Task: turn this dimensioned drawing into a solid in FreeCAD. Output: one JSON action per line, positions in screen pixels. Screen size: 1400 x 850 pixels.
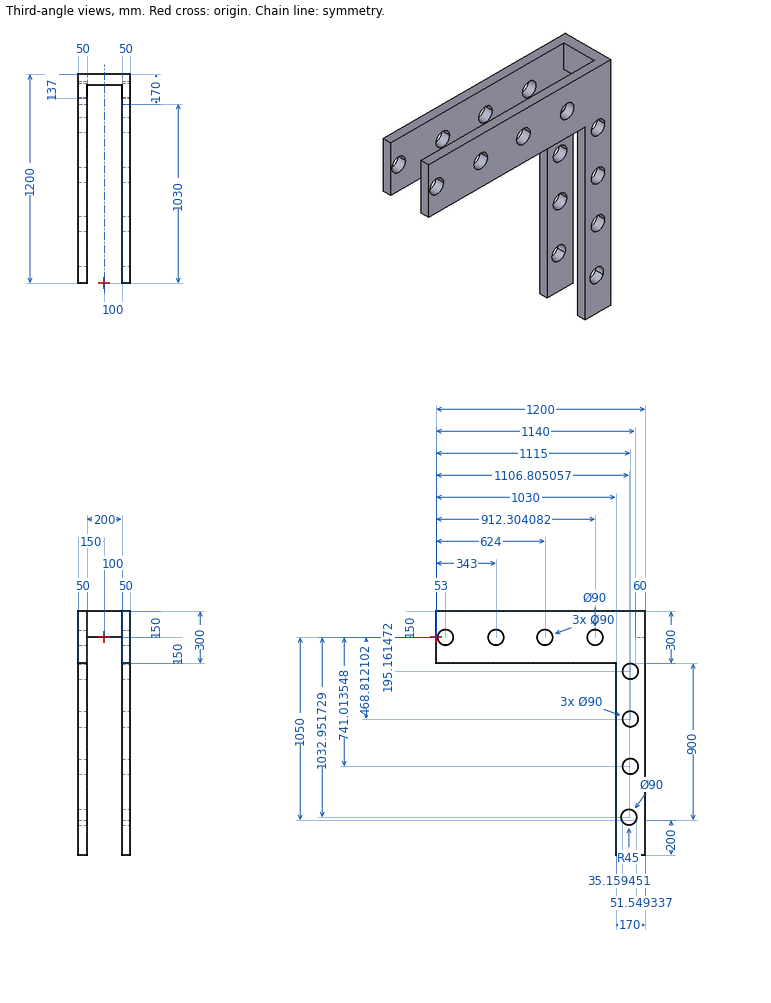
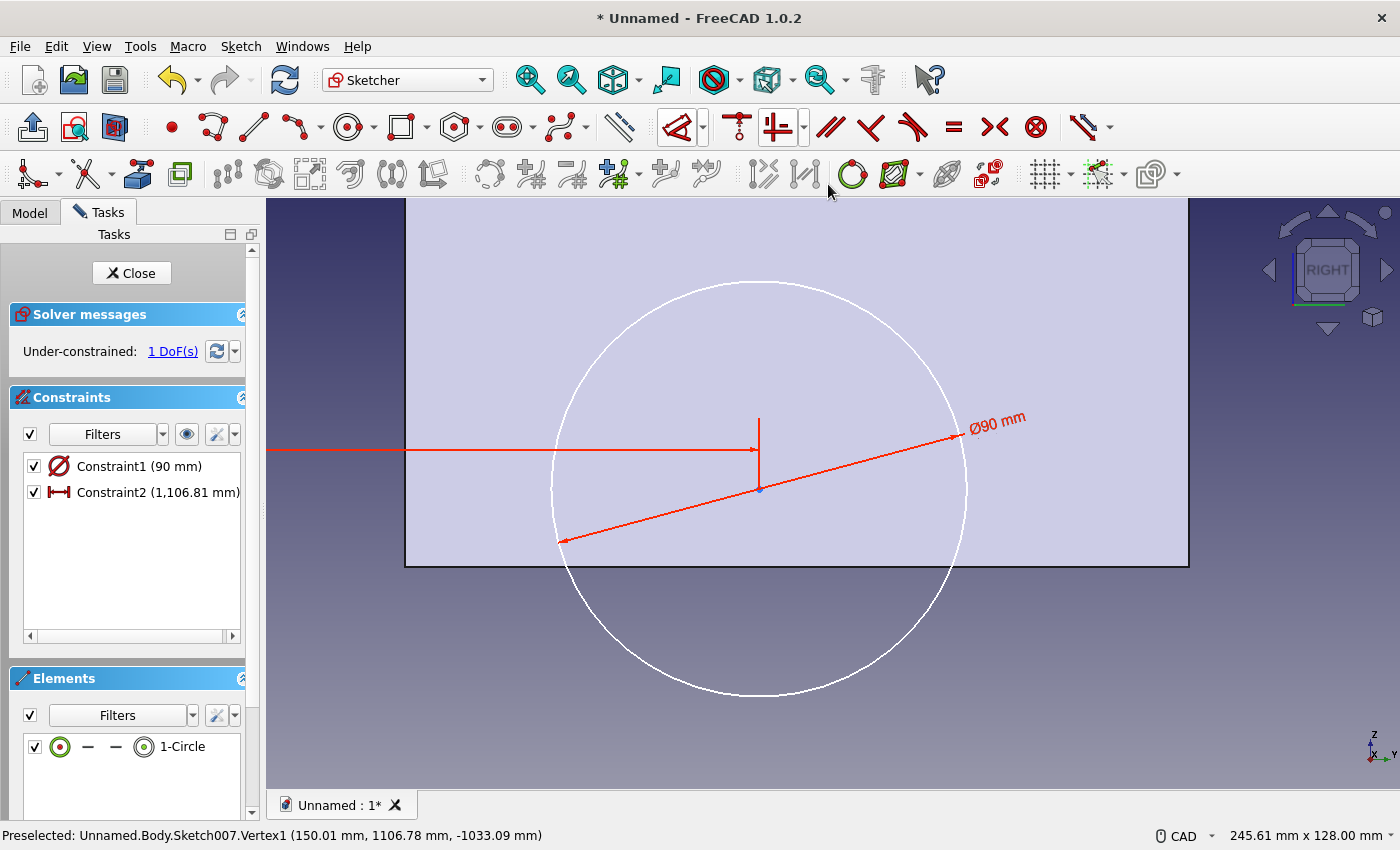
{"action": "left_click", "coordinate": [759, 489]}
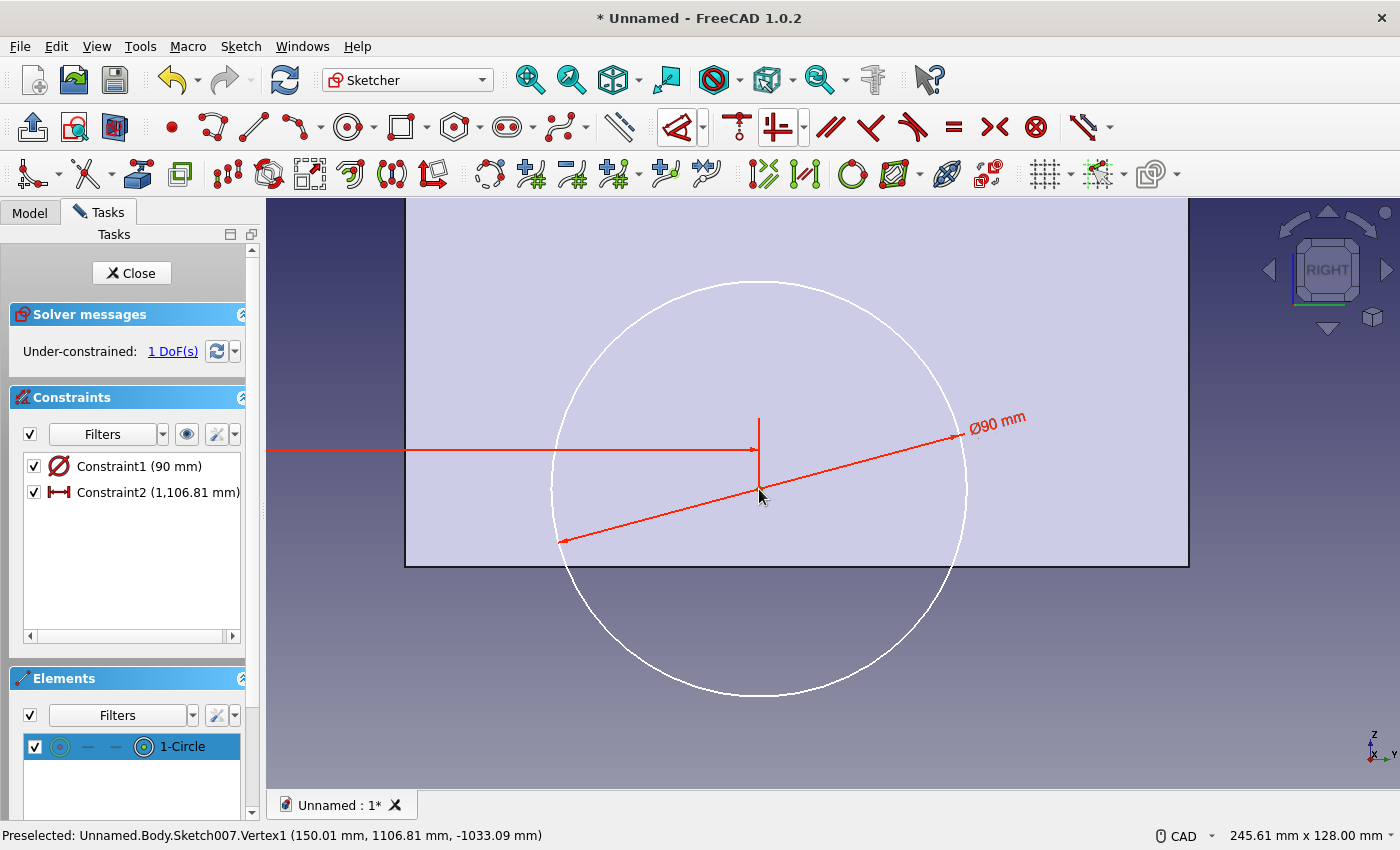
{"action": "left_click", "coordinate": [702, 128]}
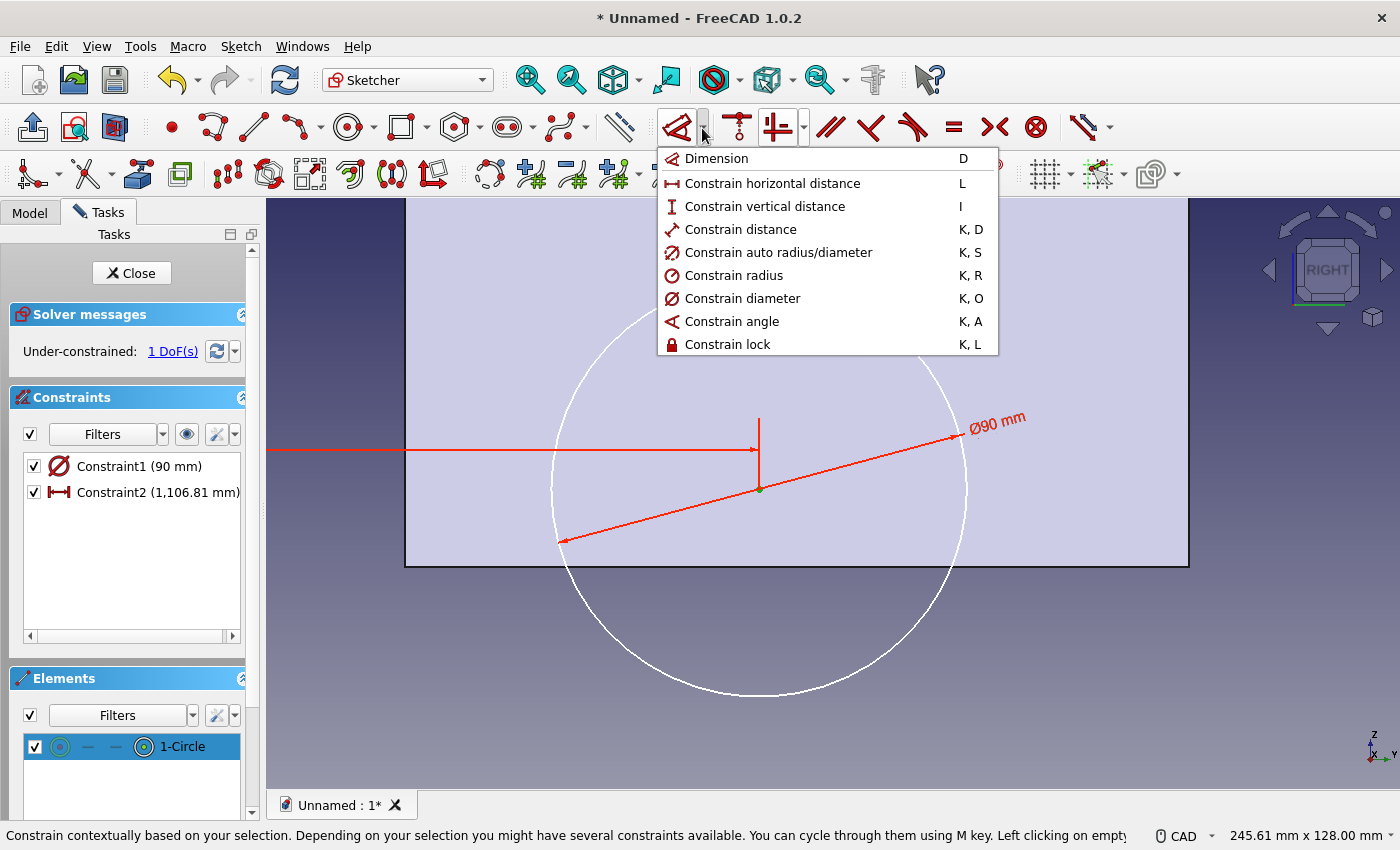
{"action": "left_click", "coordinate": [828, 206]}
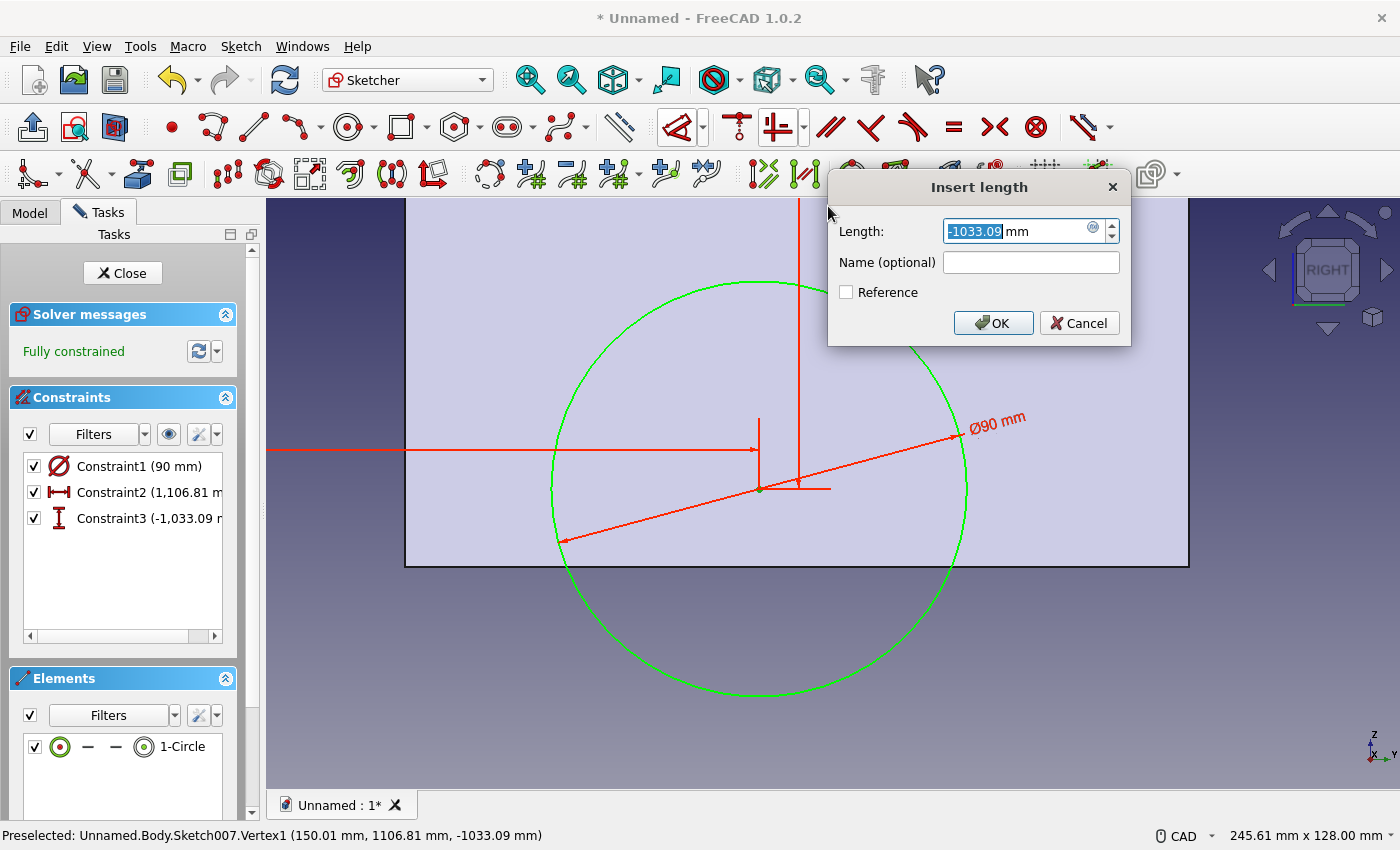
{"action": "type", "text": "-1032.951729"}
{"action": "key", "text": "Return"}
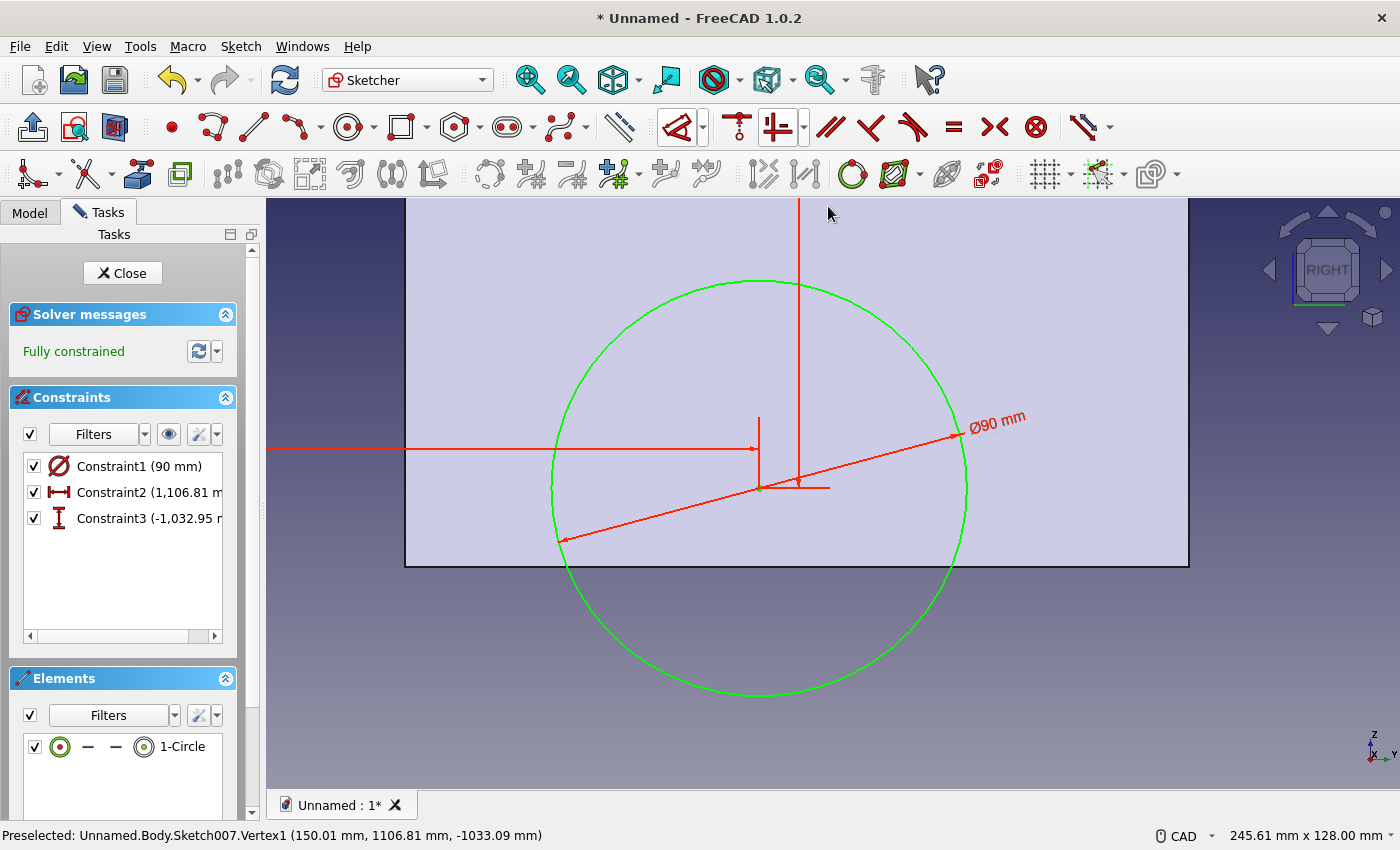
{"action": "left_click", "coordinate": [123, 273]}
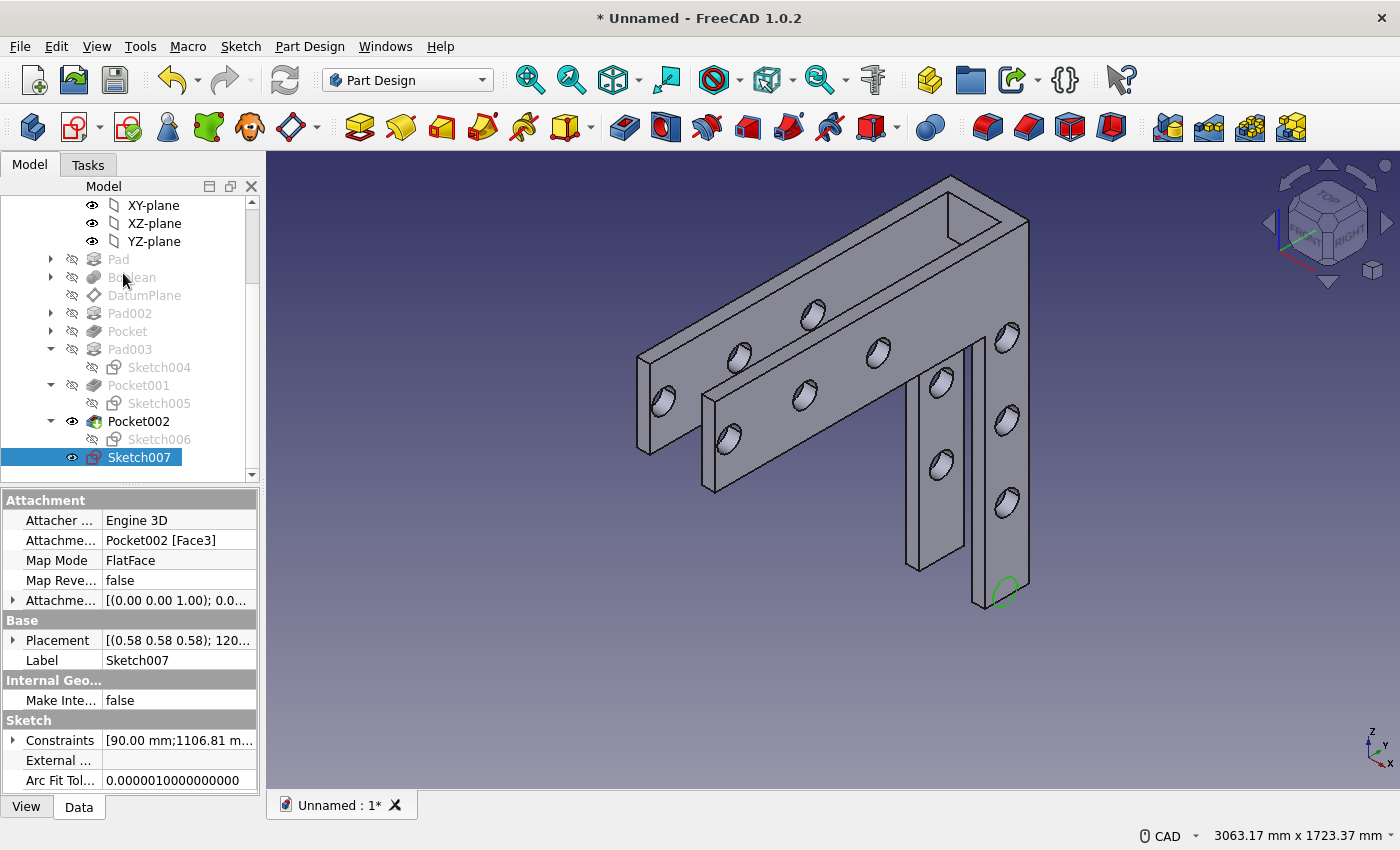
{"action": "left_click", "coordinate": [625, 128]}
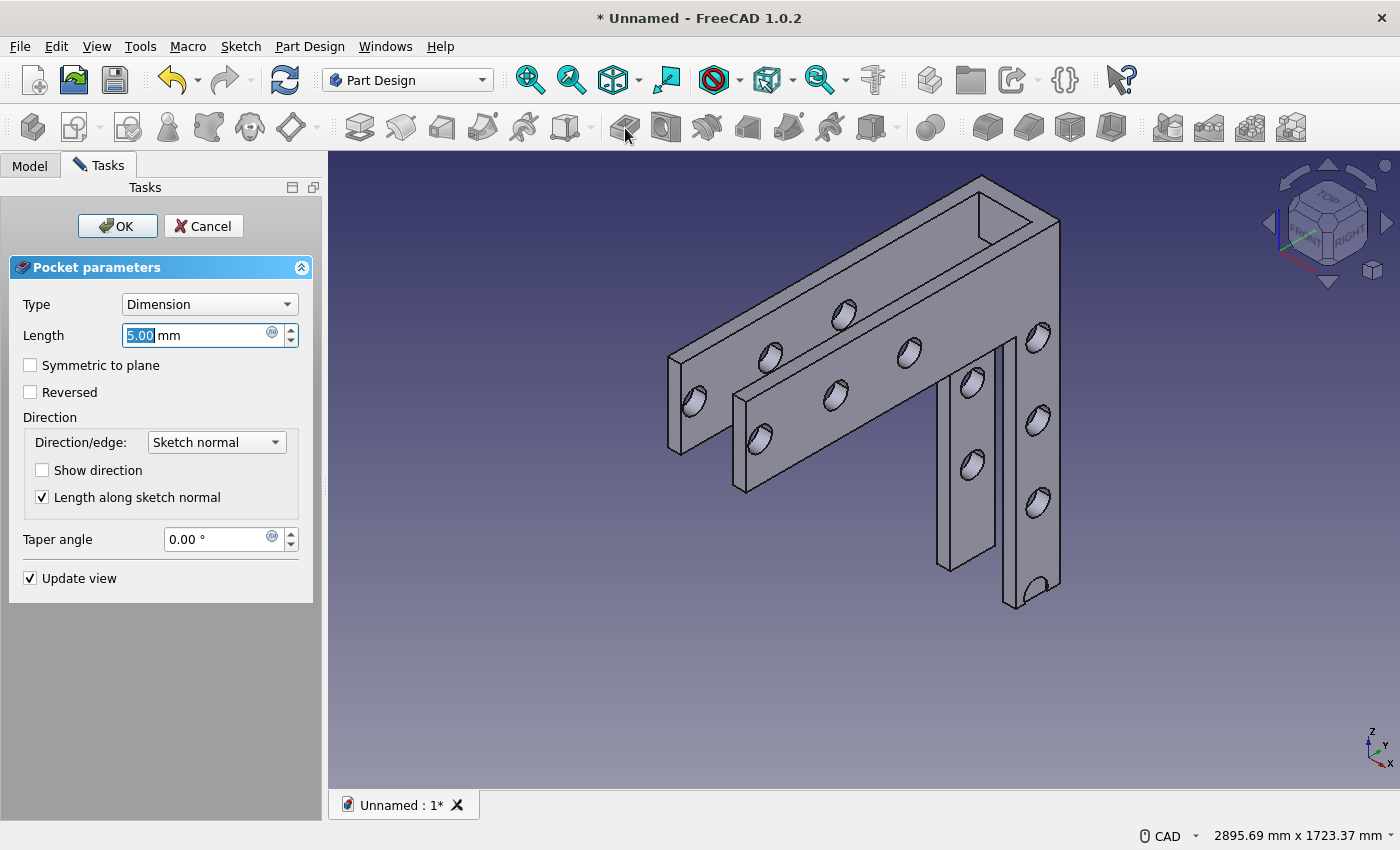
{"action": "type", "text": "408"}
{"action": "key", "text": "Tab"}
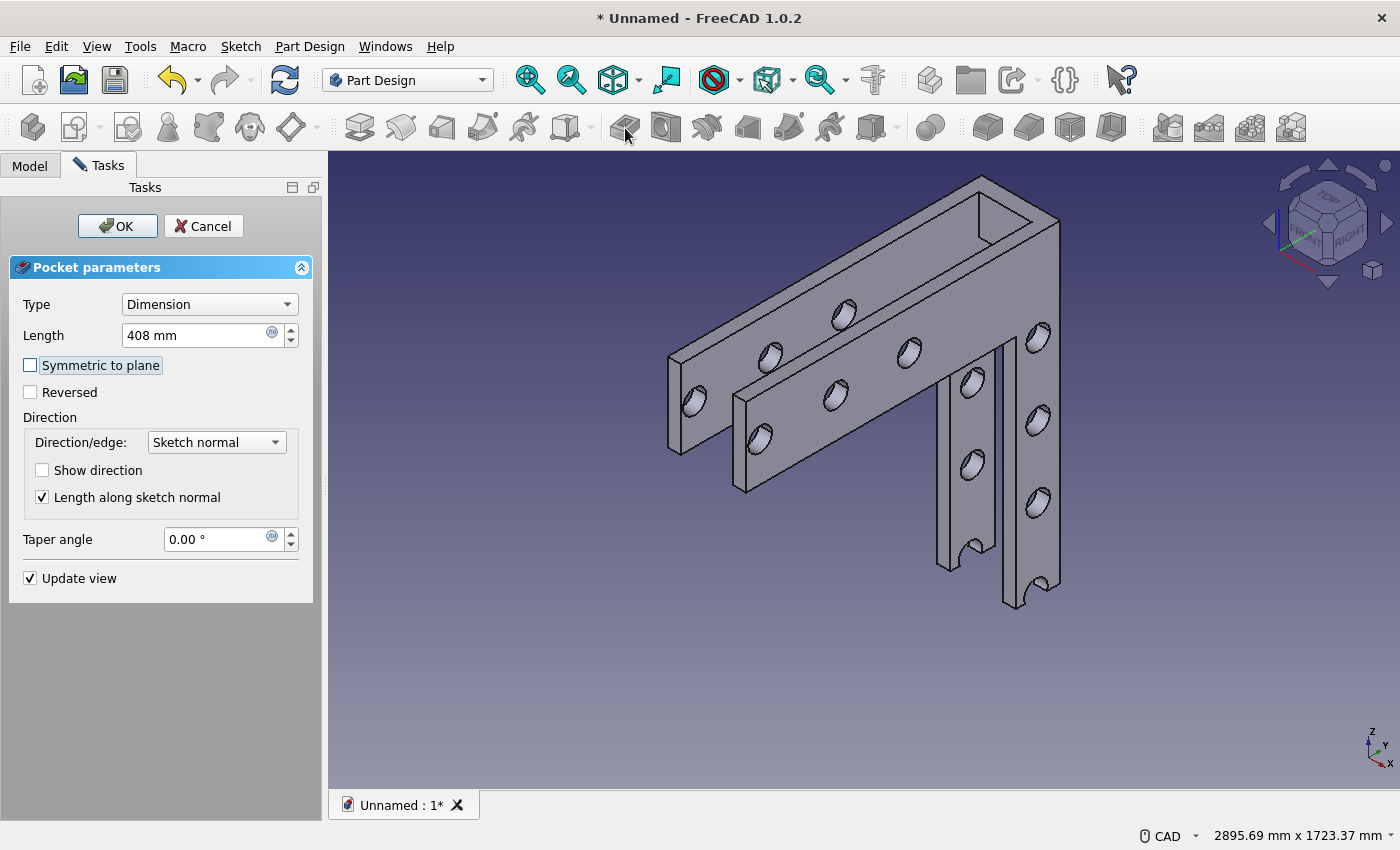
{"action": "left_click", "coordinate": [118, 226]}